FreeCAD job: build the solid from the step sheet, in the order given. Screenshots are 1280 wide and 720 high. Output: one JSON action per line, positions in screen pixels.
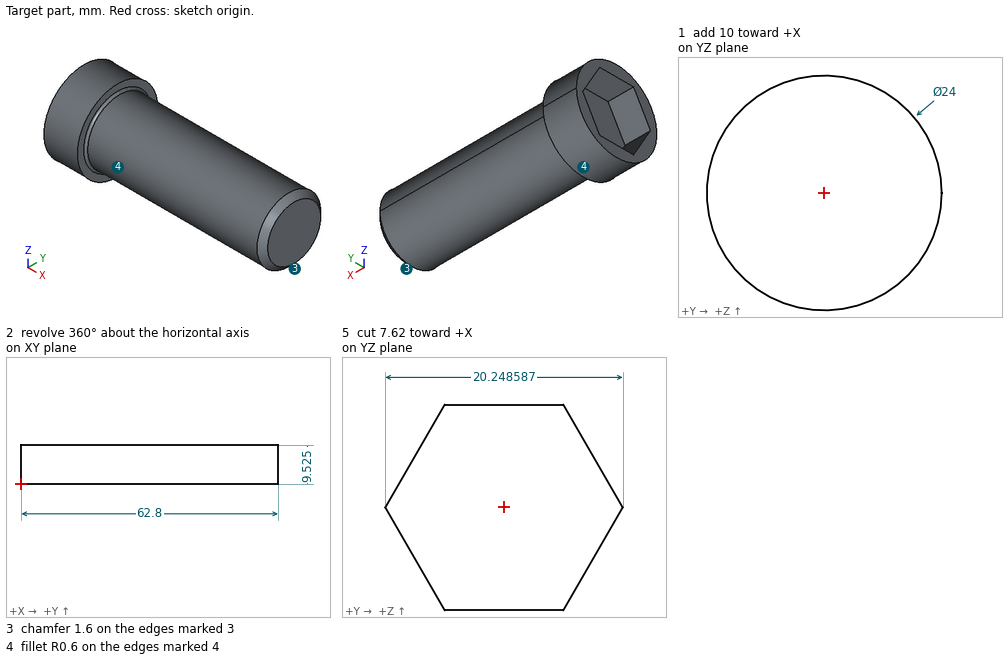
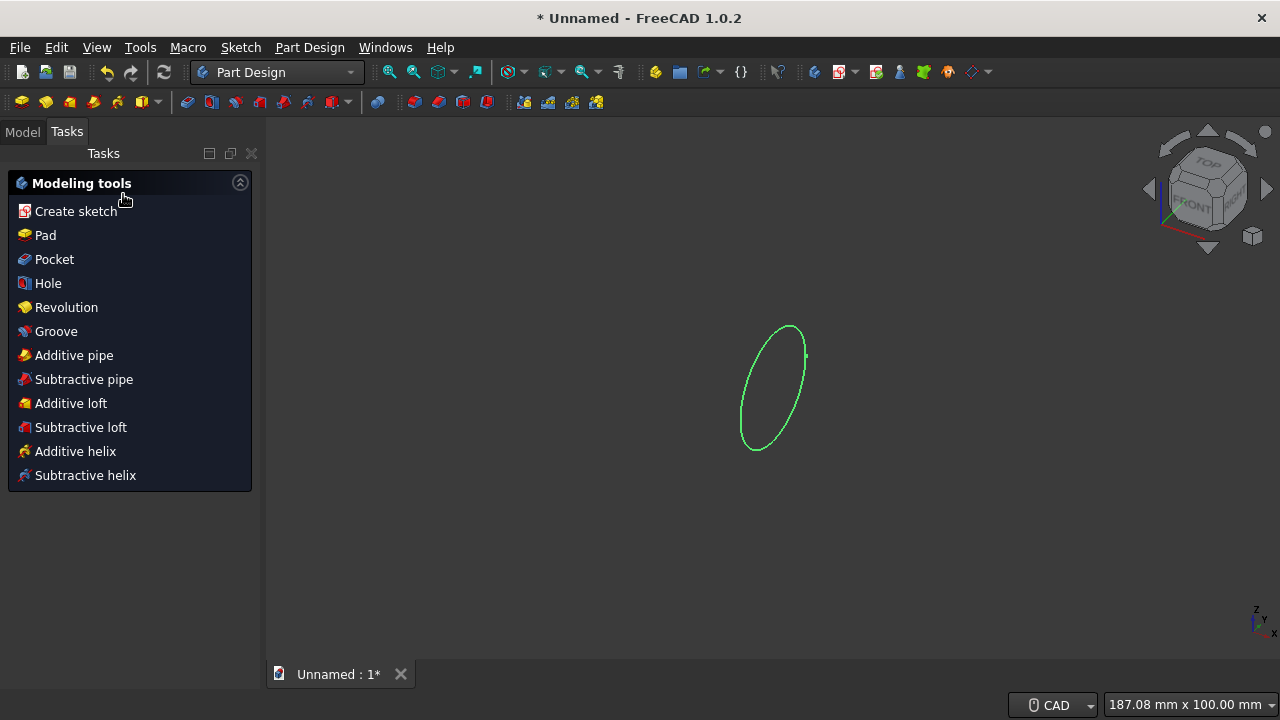
{"action": "left_click", "coordinate": [22, 102]}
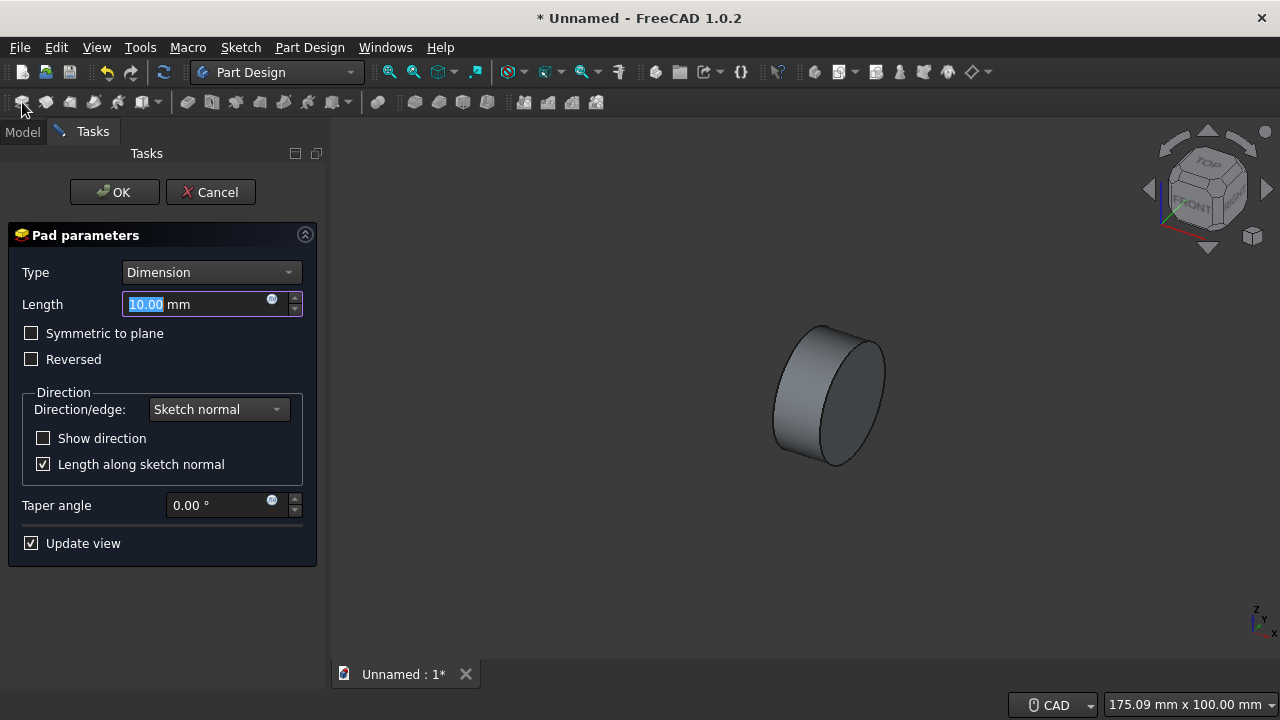
{"action": "type", "text": "10"}
{"action": "key", "text": "Tab"}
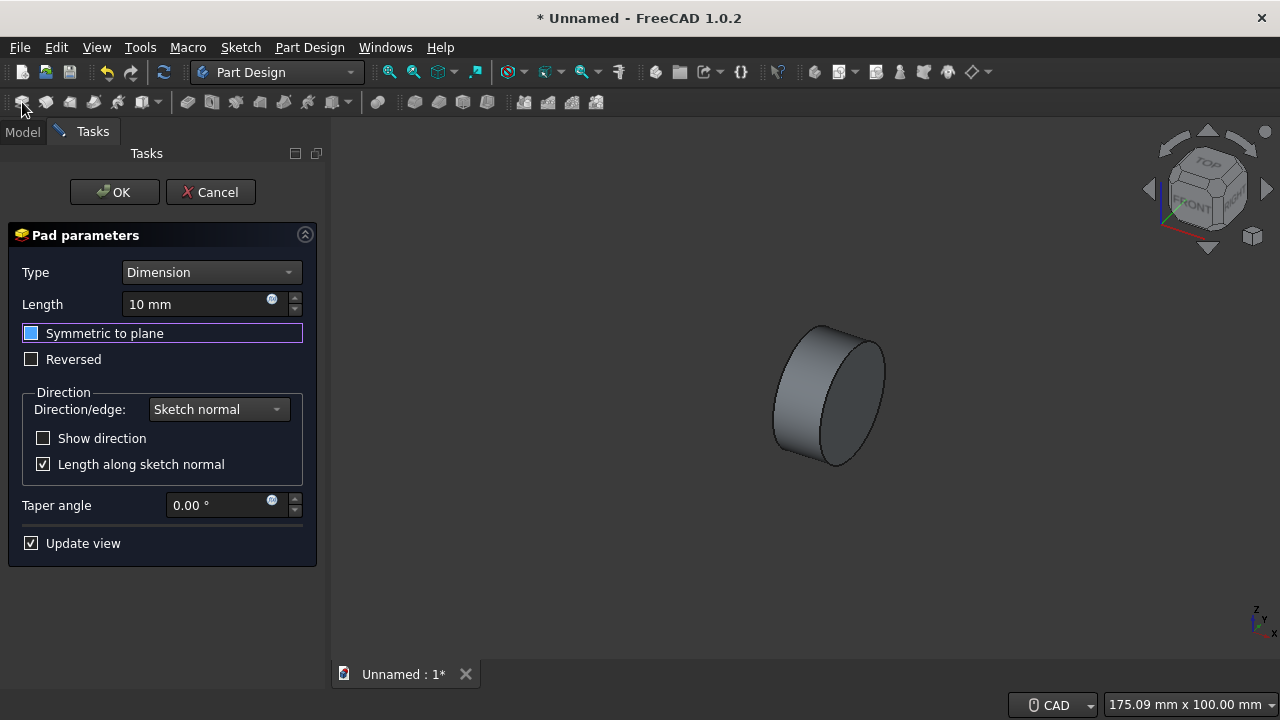
{"action": "left_click", "coordinate": [115, 192]}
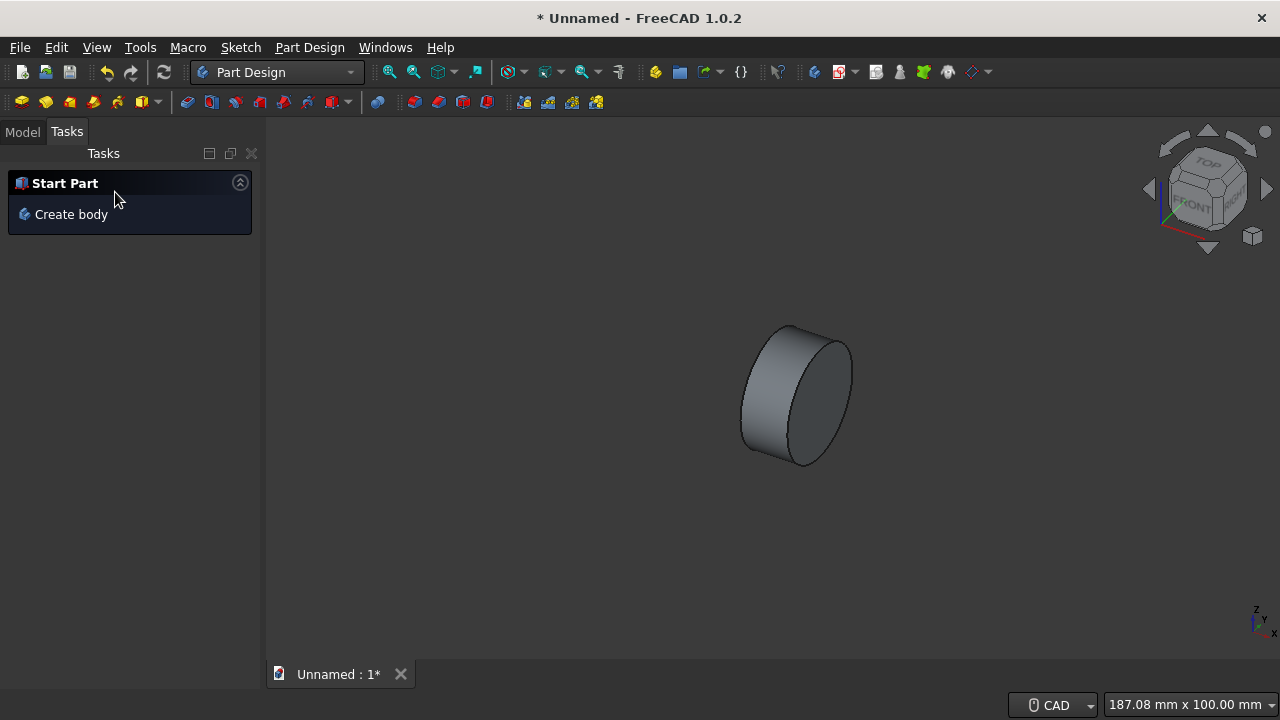
{"action": "left_click", "coordinate": [390, 72]}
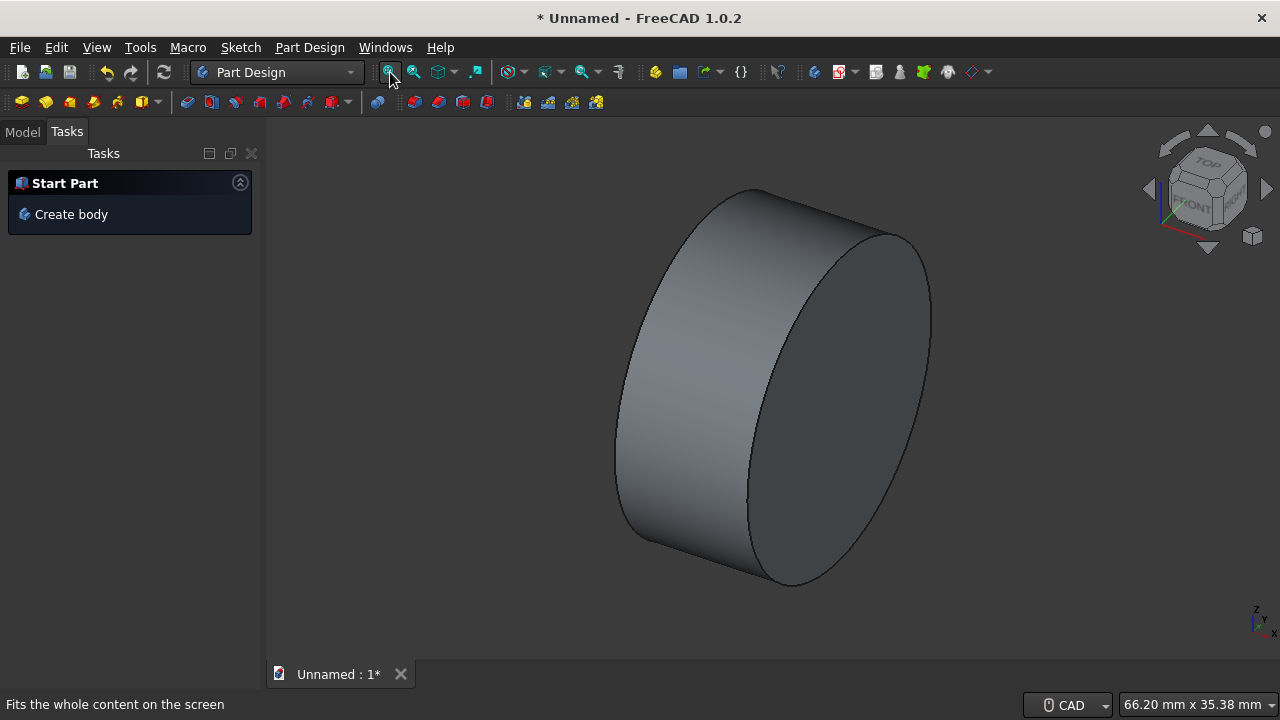
{"action": "left_click", "coordinate": [840, 72]}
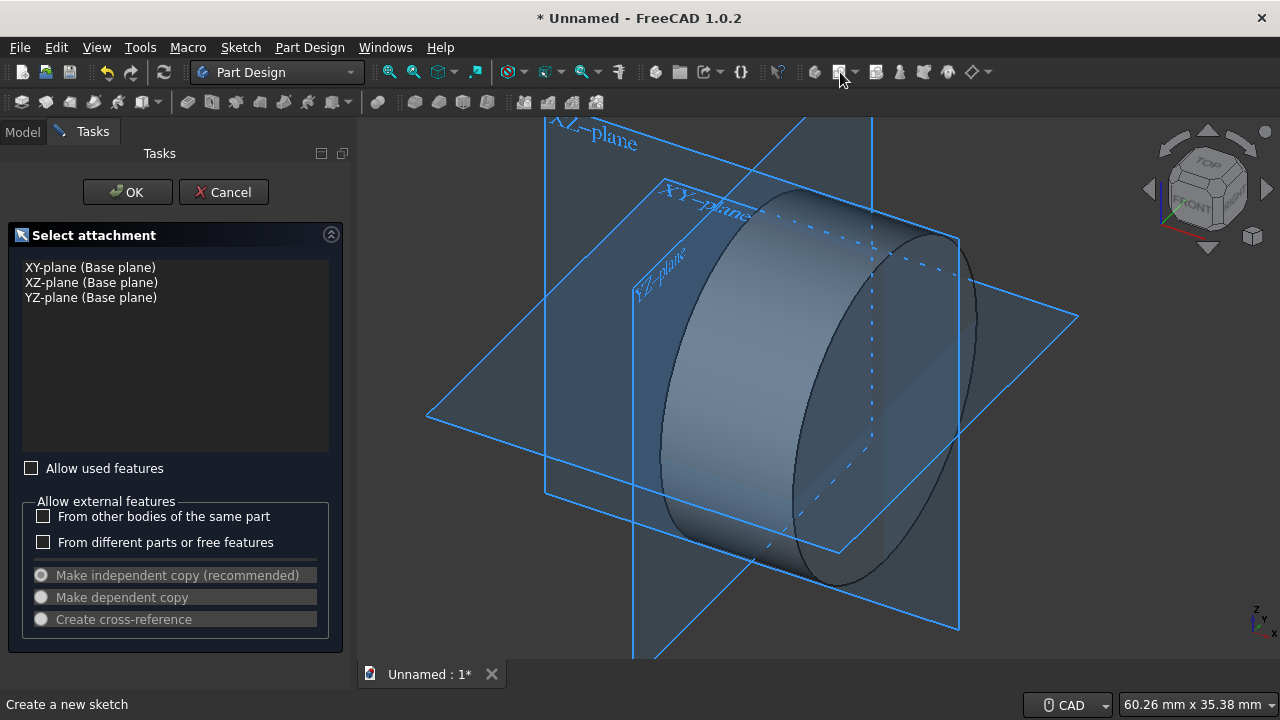
{"action": "left_click", "coordinate": [82, 268]}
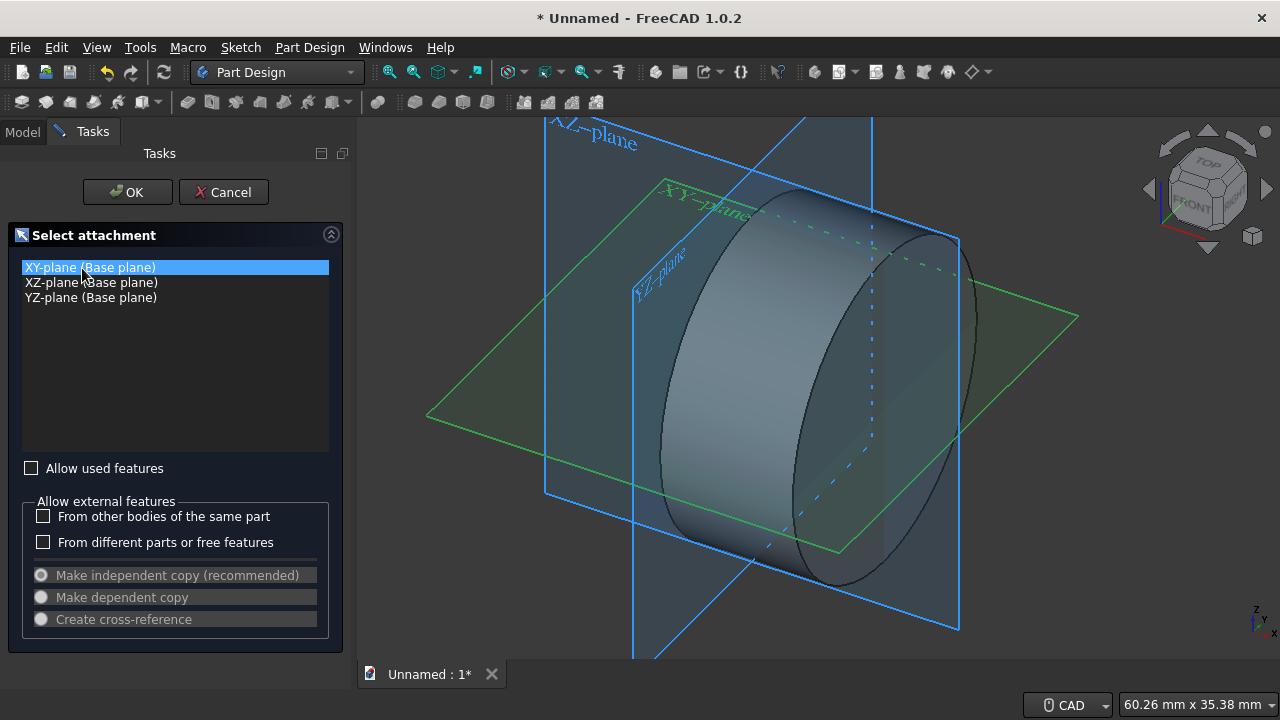
{"action": "left_click", "coordinate": [128, 192]}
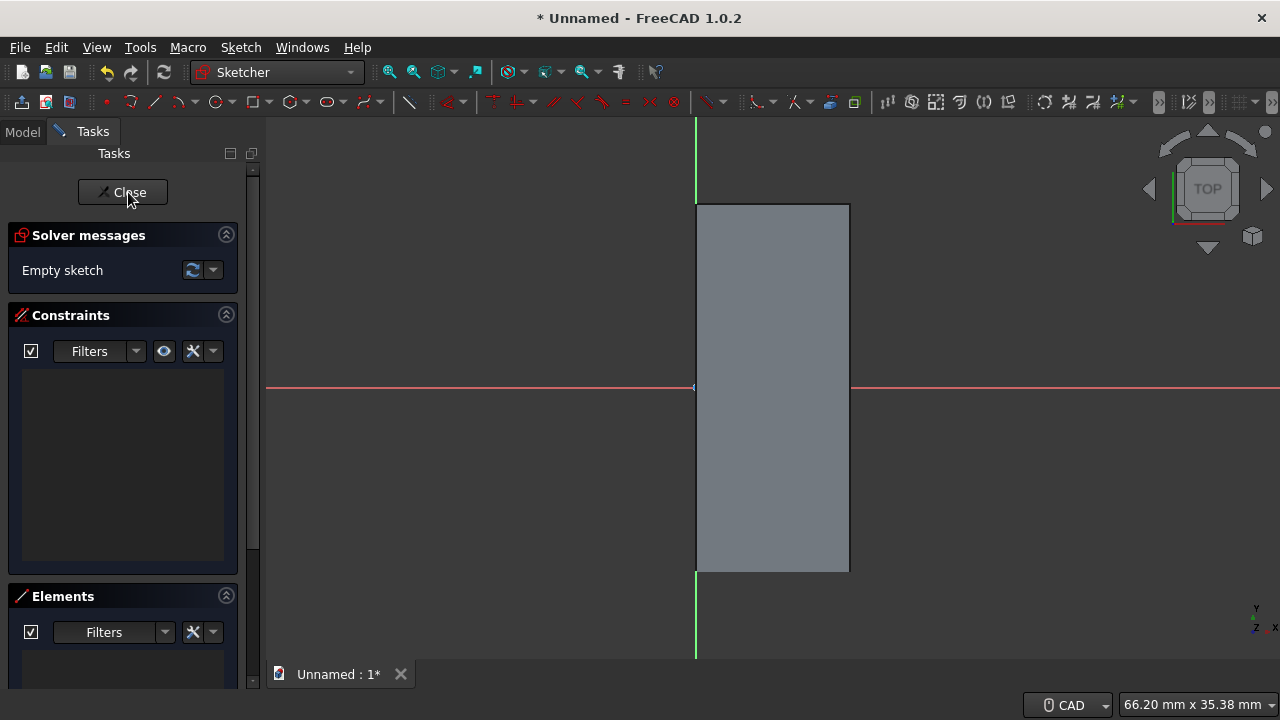
{"action": "left_click", "coordinate": [70, 102]}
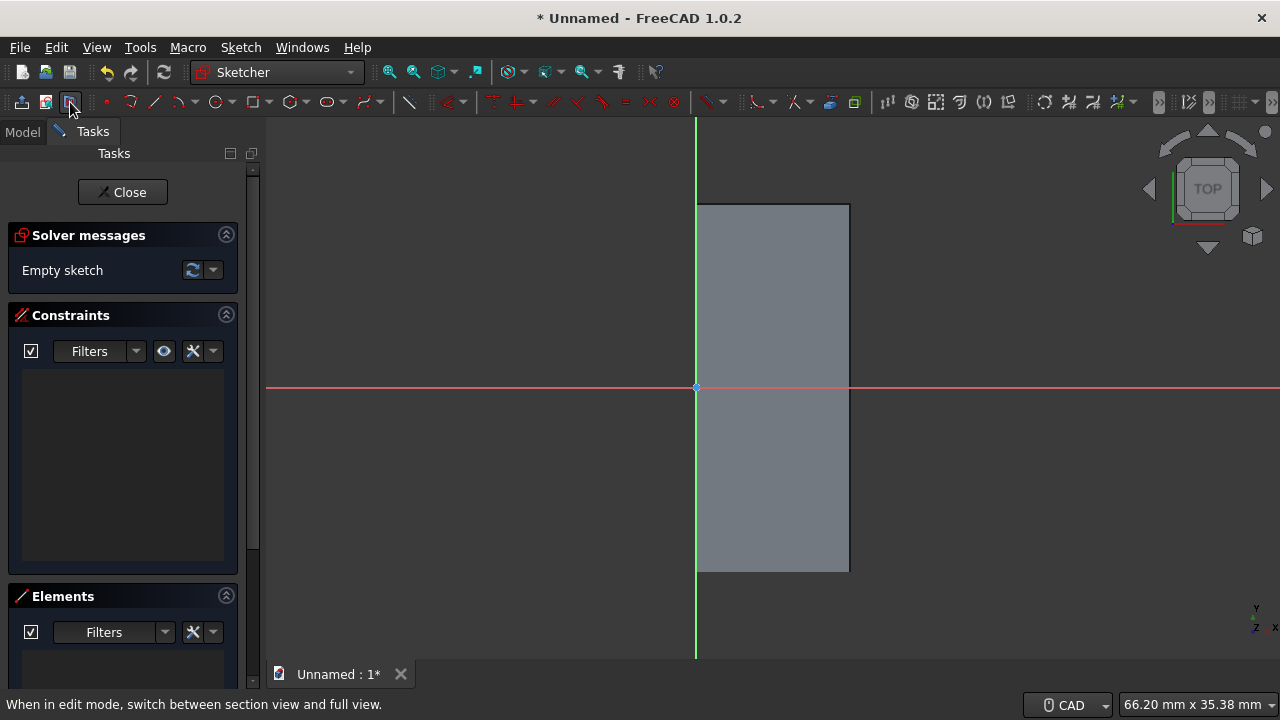
{"action": "scroll", "coordinate": [294, 477], "scroll_direction": "down", "scroll_amount": 3}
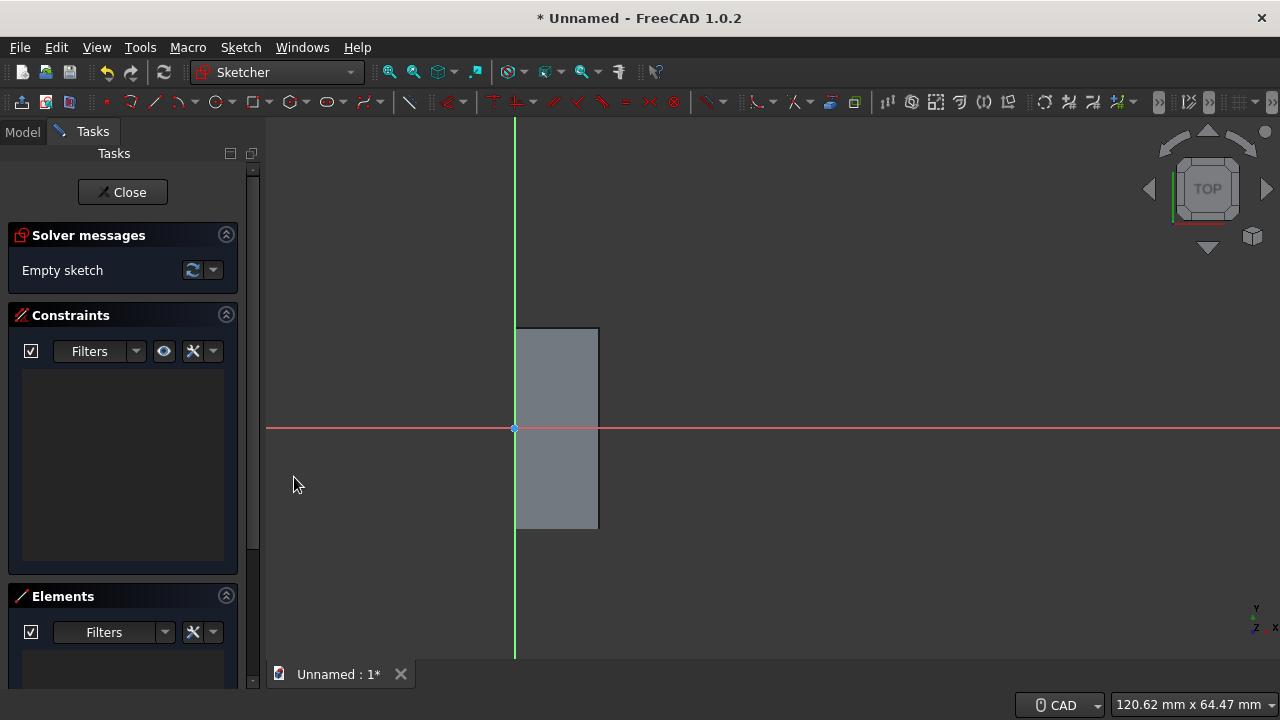
{"action": "left_click", "coordinate": [254, 102]}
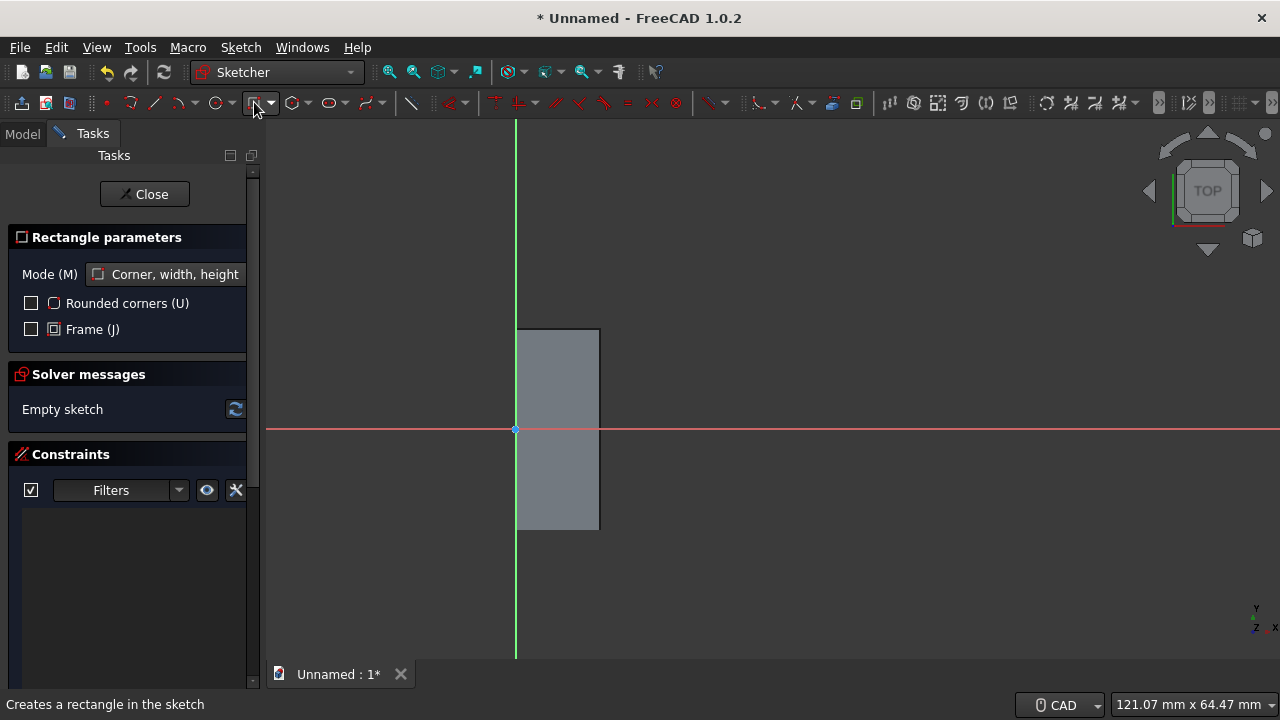
{"action": "left_click", "coordinate": [516, 429]}
{"action": "left_click", "coordinate": [1042, 350]}
{"action": "key", "text": "Escape"}